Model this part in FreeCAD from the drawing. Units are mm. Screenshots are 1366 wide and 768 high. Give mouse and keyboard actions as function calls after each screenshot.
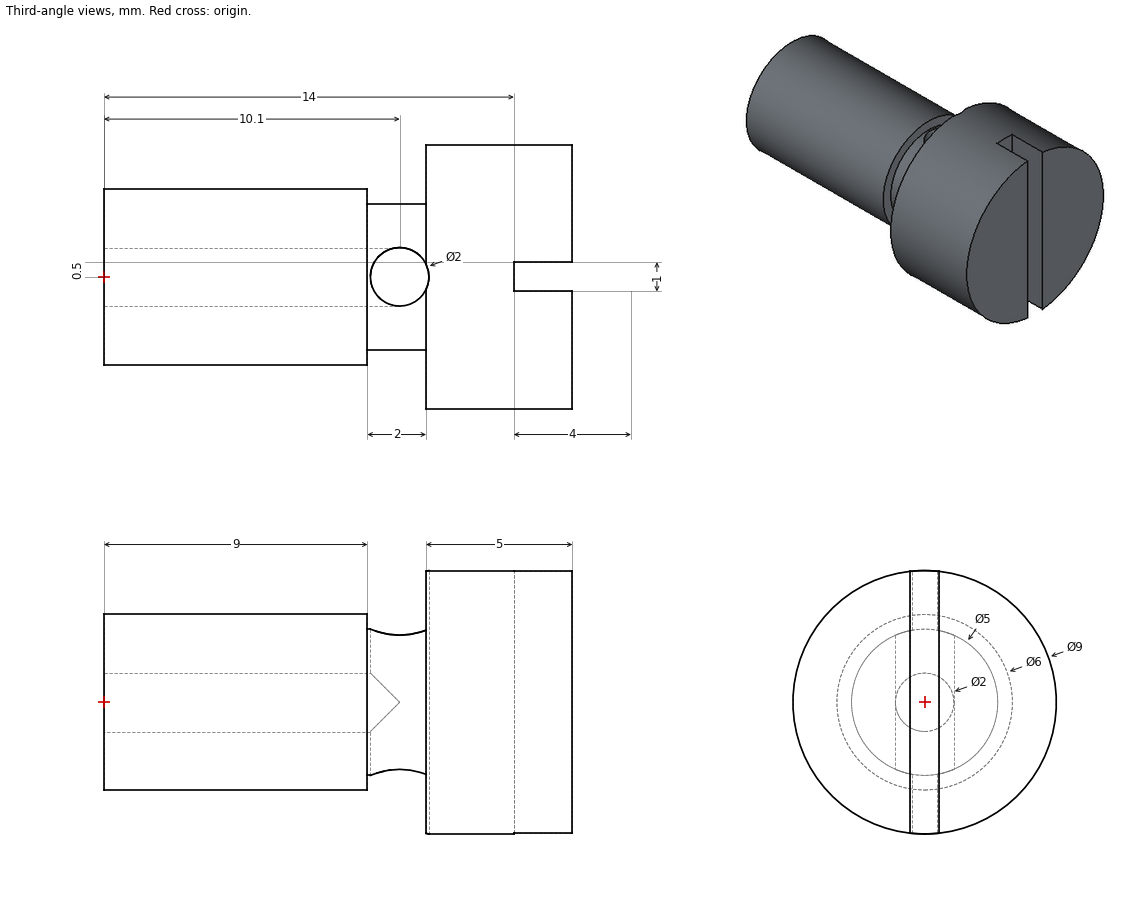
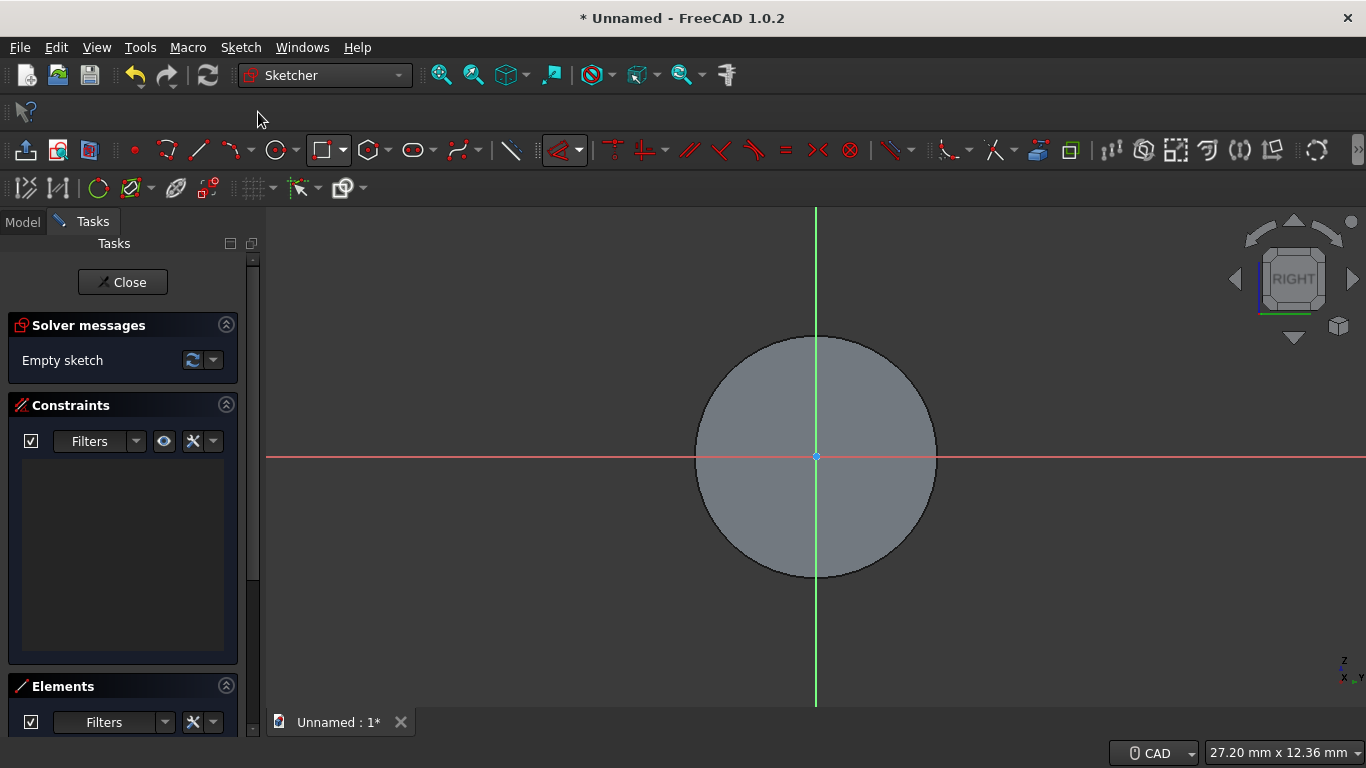
scroll(955, 457, up, 2)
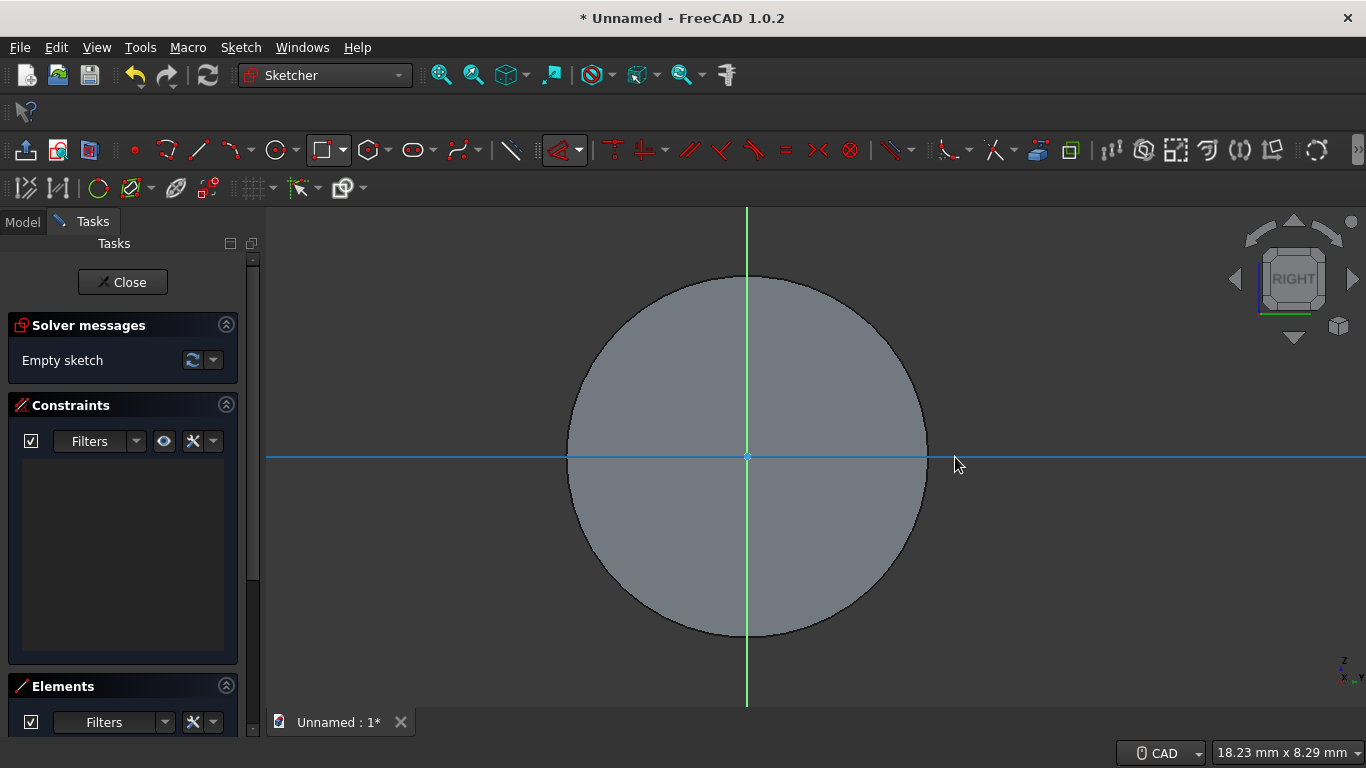
click(276, 150)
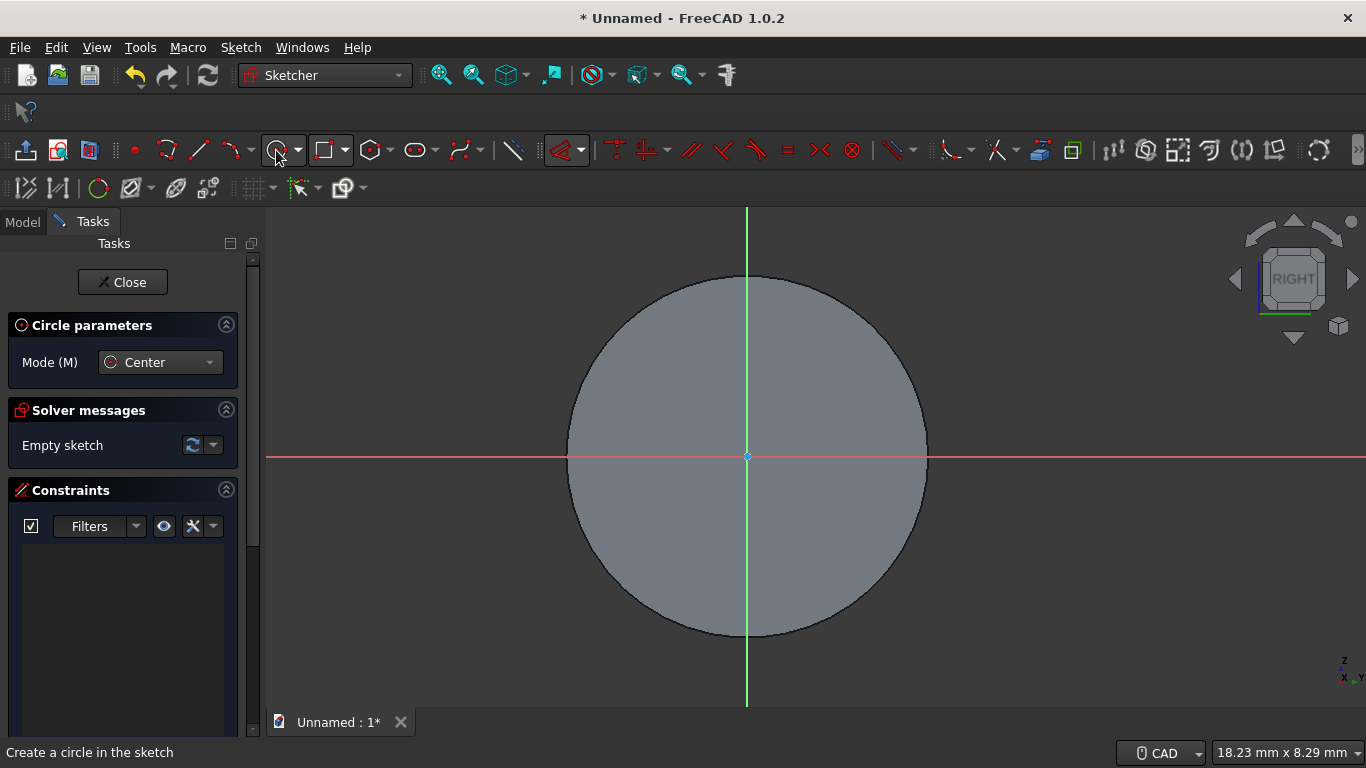
click(747, 457)
click(854, 350)
key(Escape)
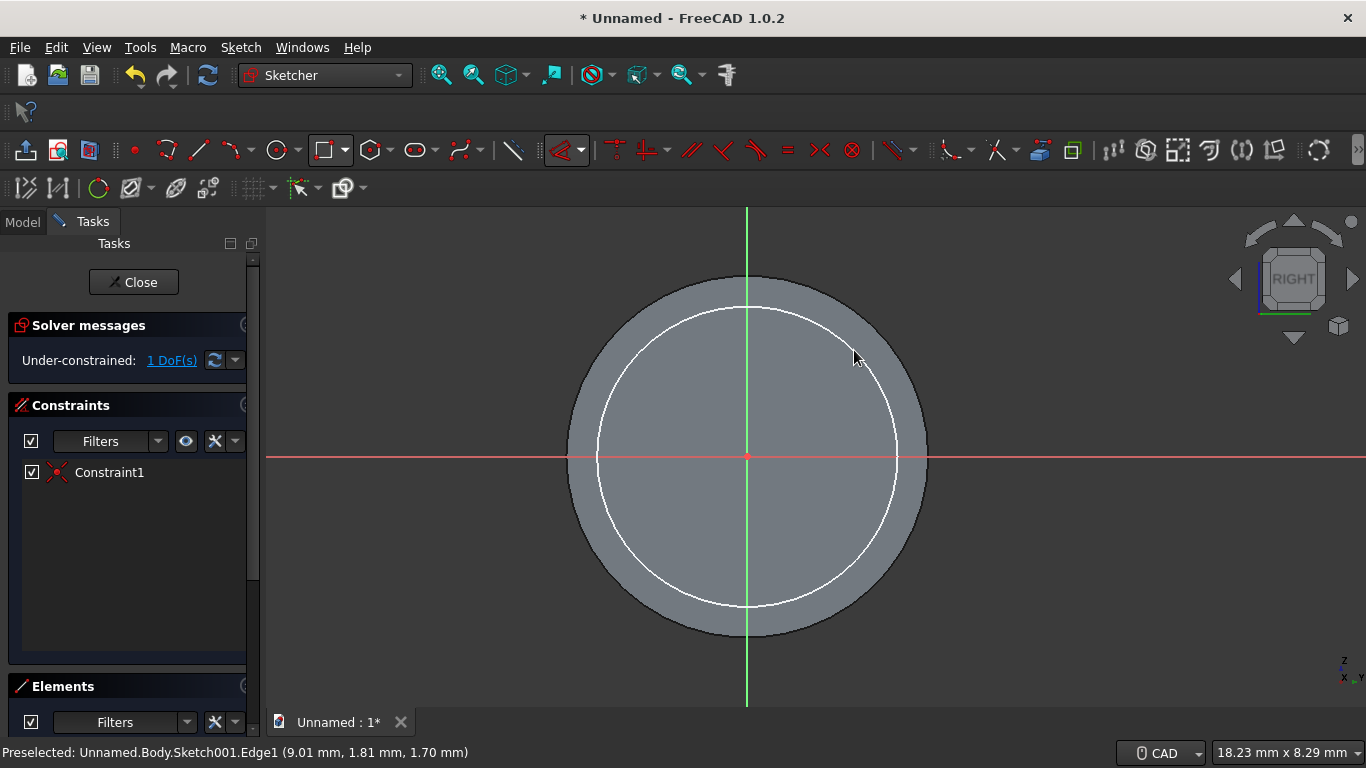
click(853, 350)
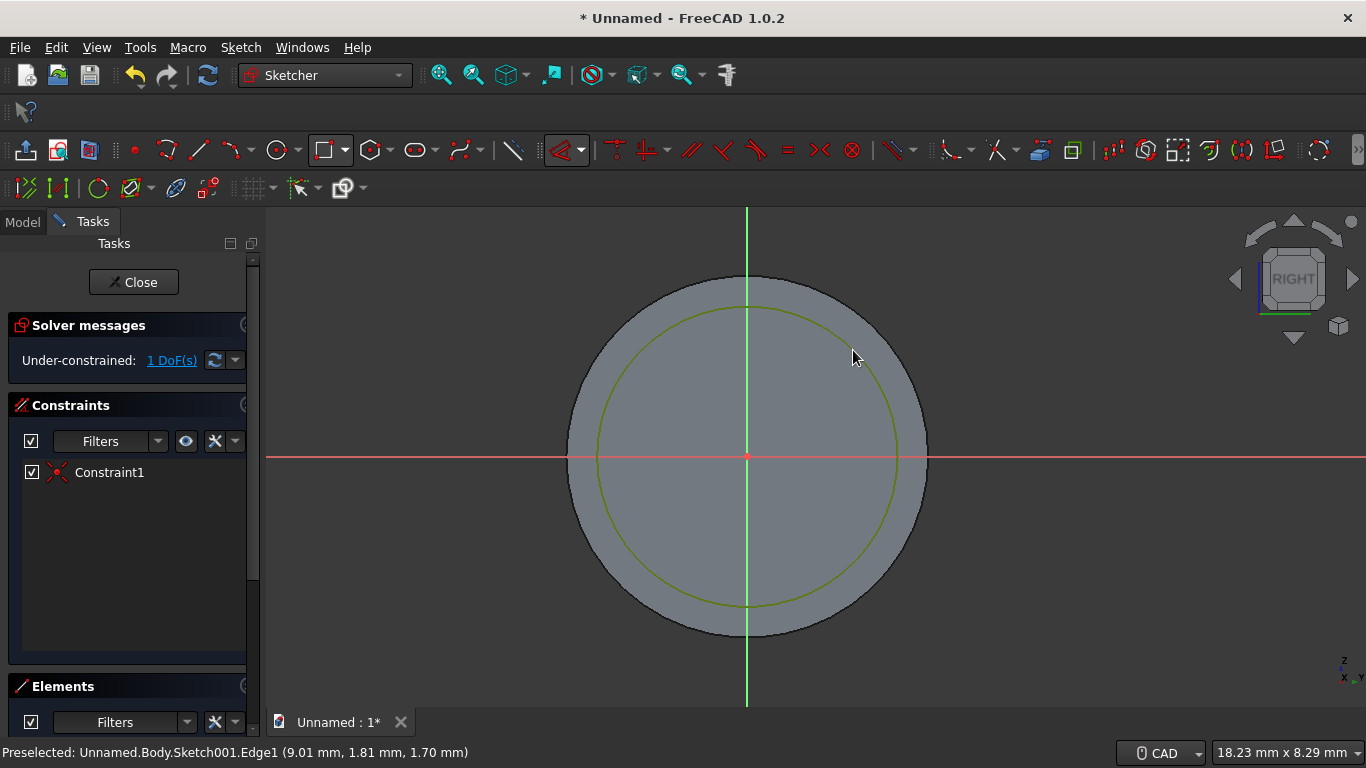
key(k)
key(o)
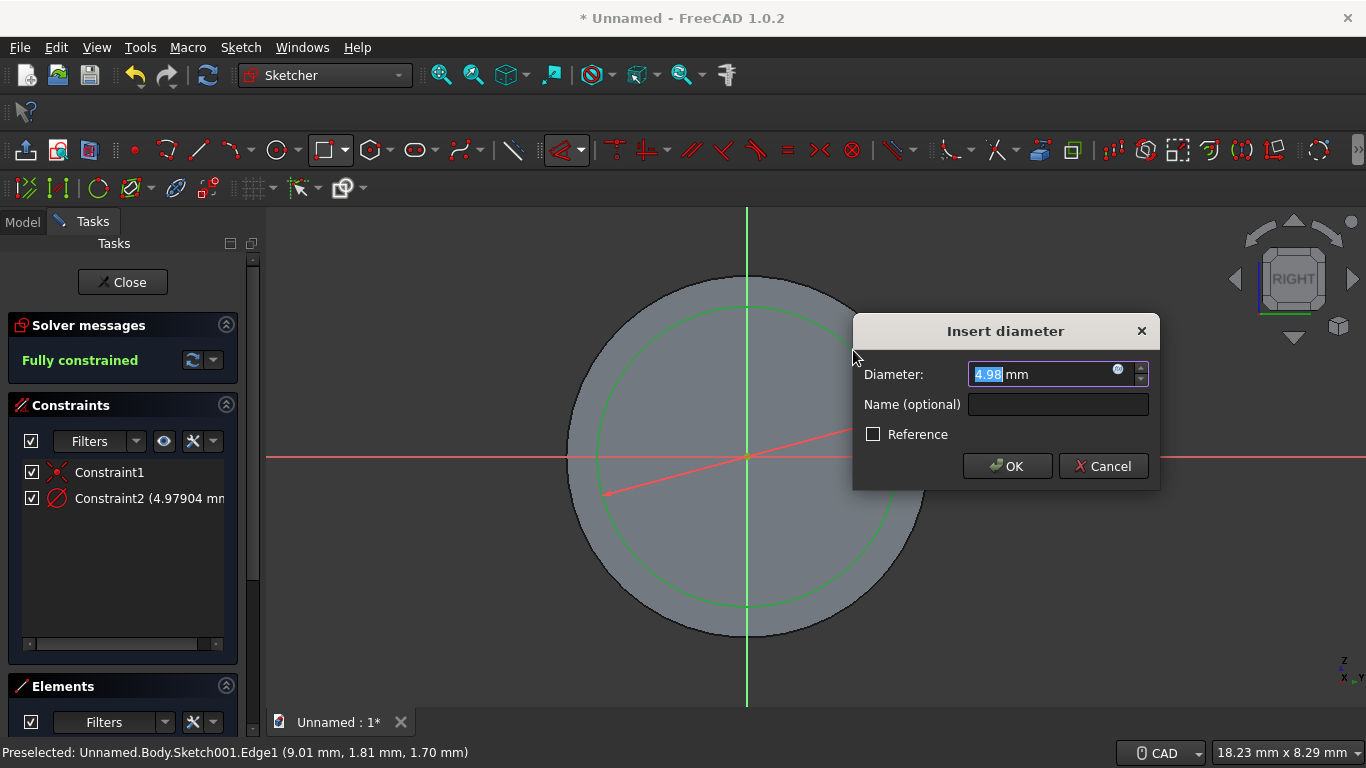
text(5)
key(Return)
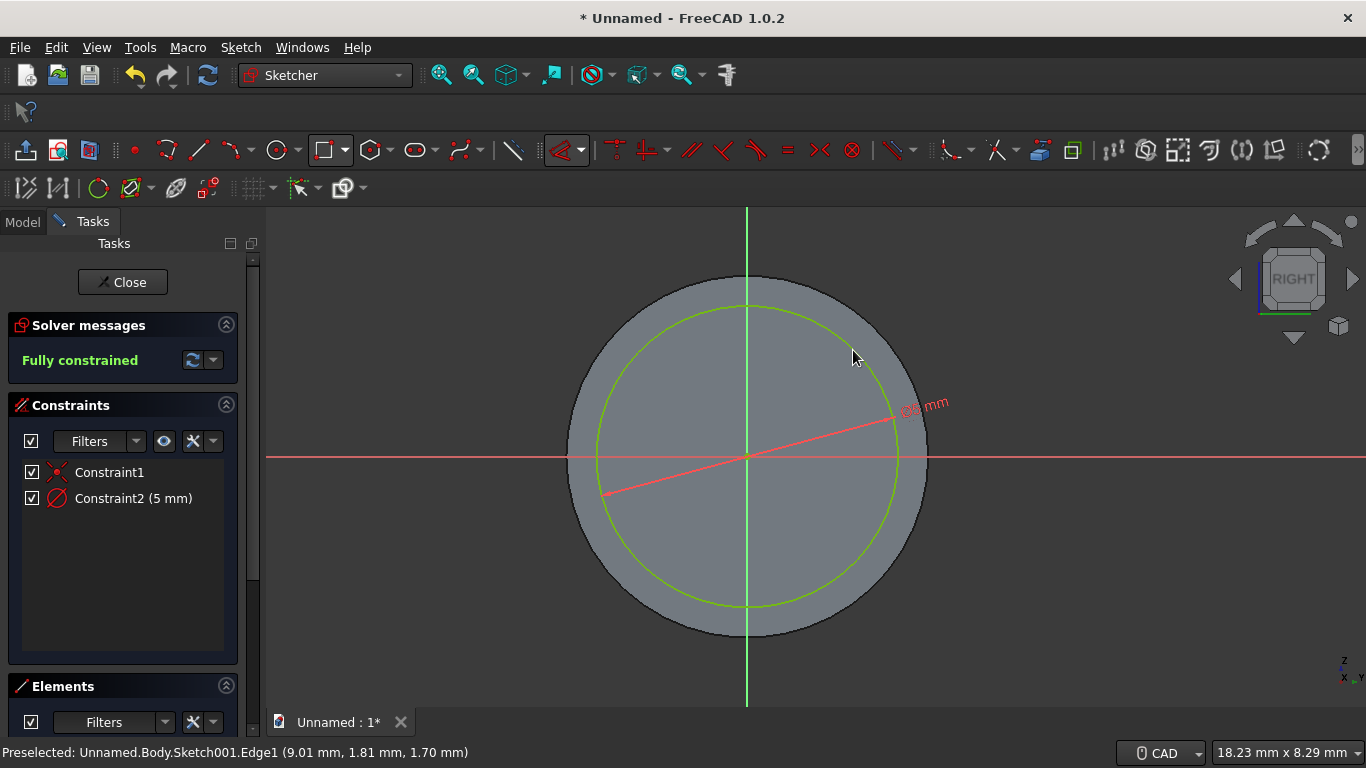
click(123, 282)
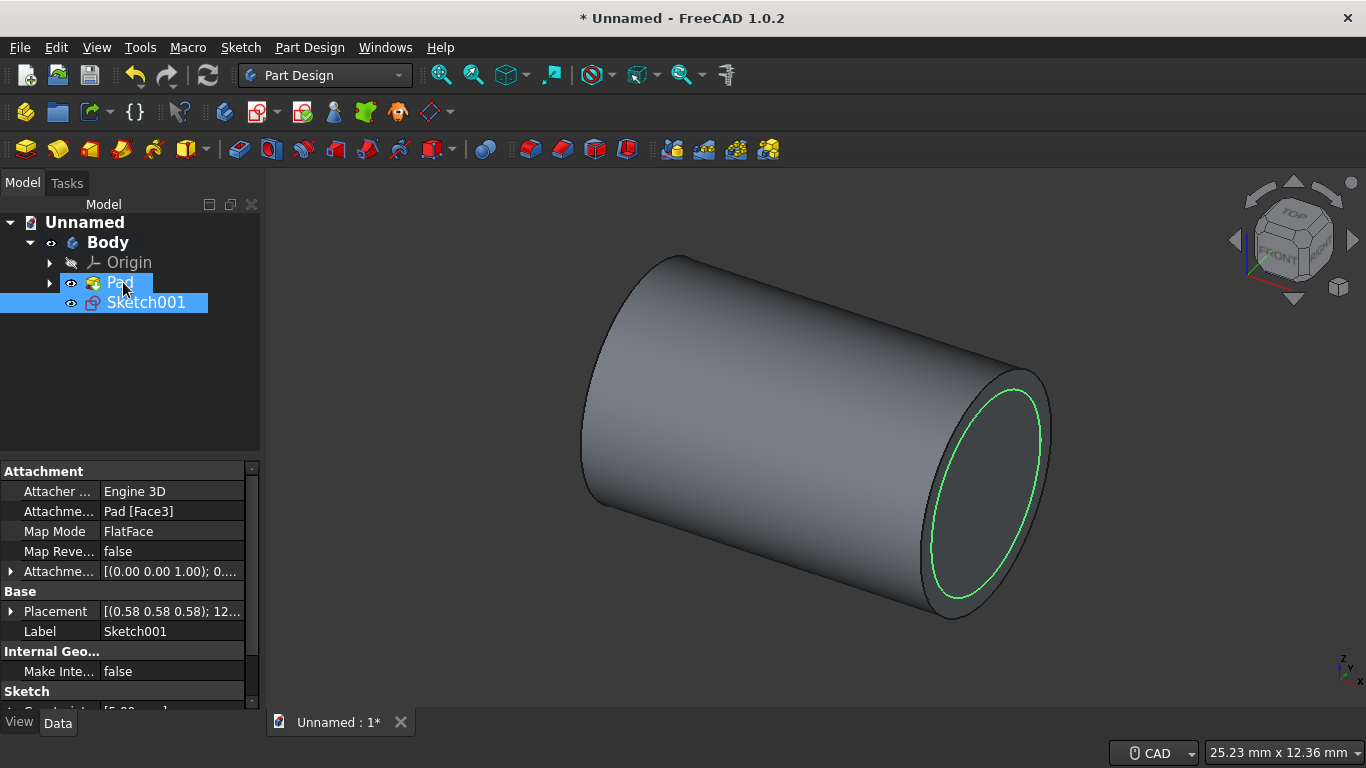
click(26, 150)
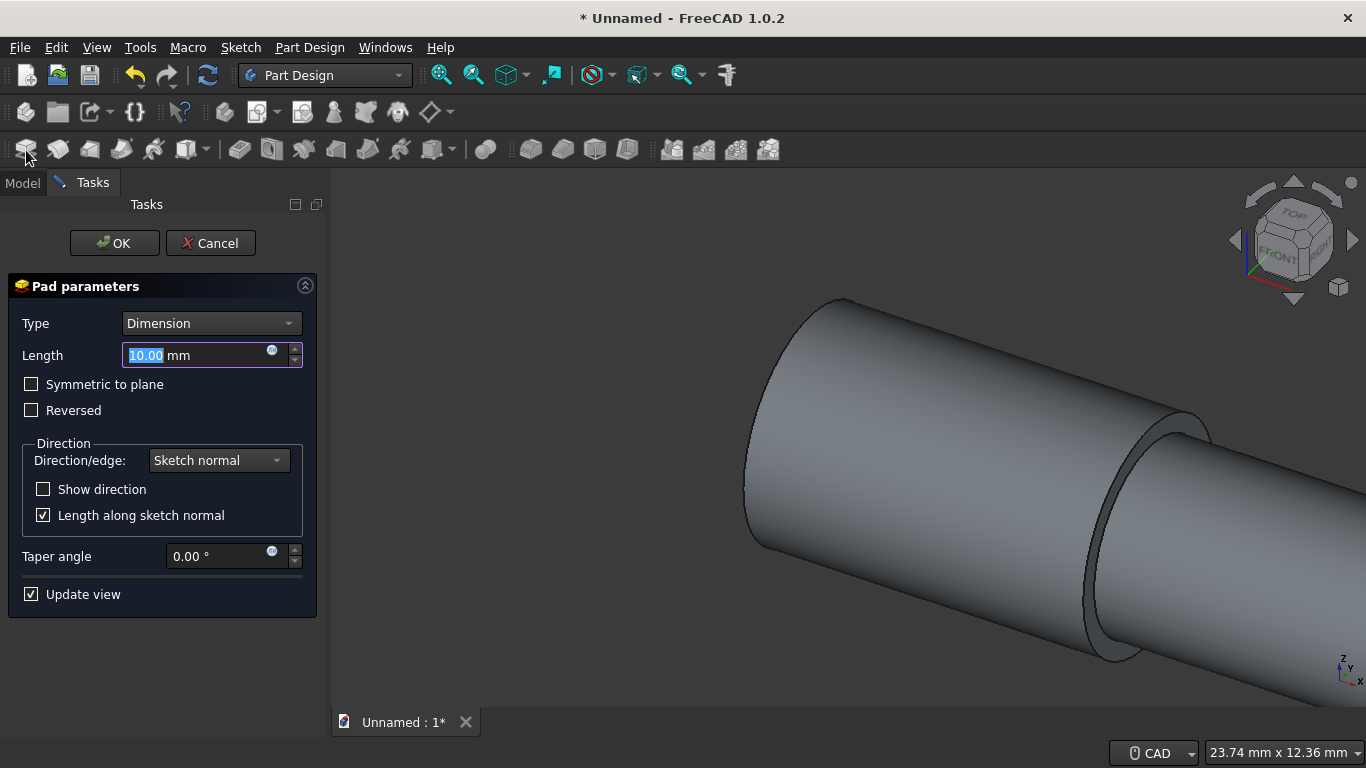
text(2)
key(Tab)